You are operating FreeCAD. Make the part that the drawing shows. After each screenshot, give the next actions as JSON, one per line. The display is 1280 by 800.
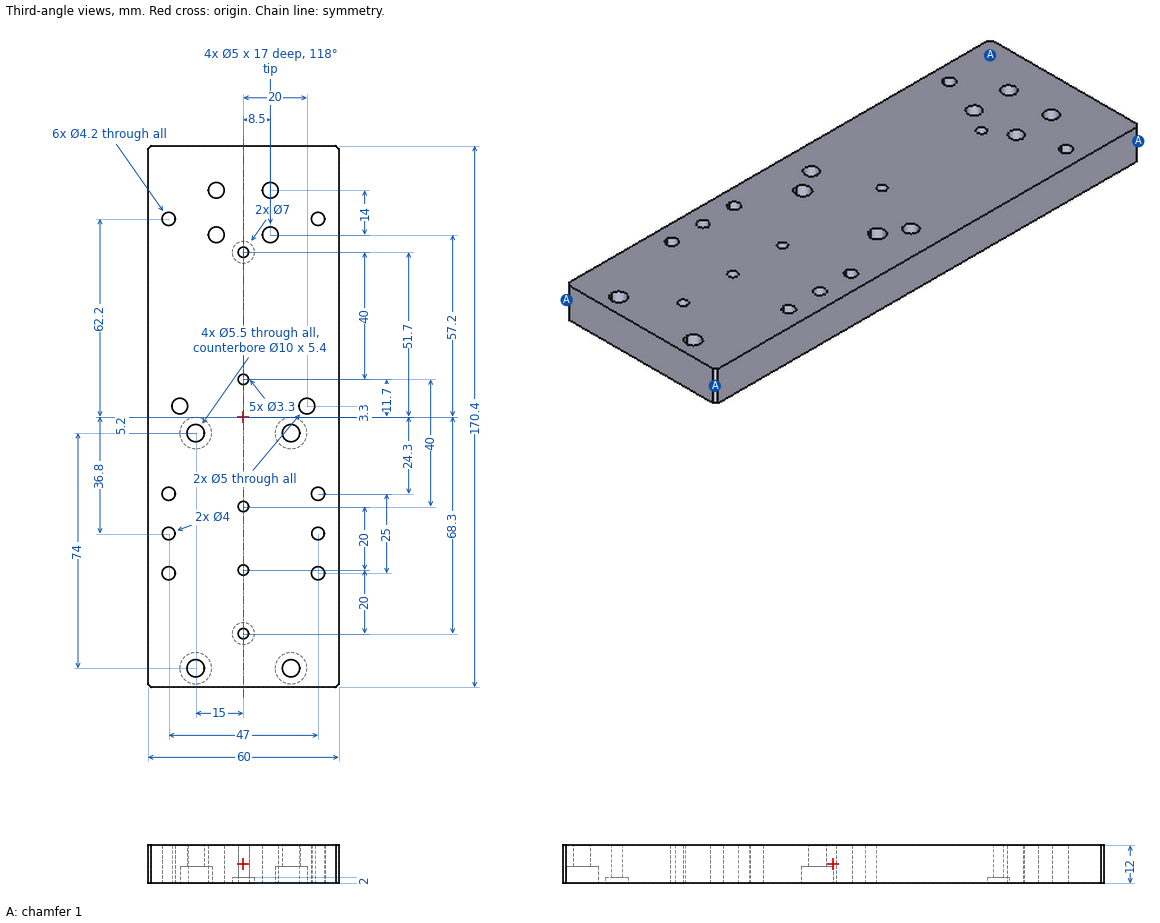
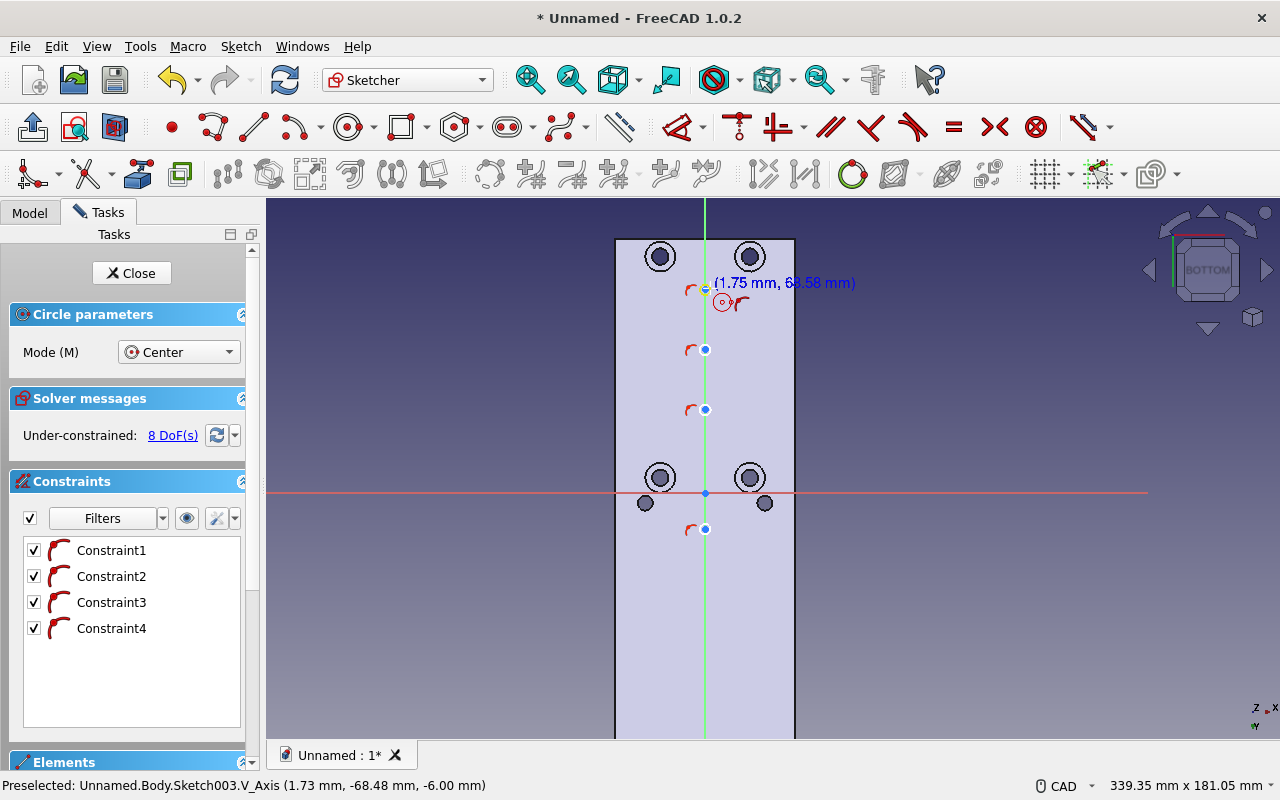
{"action": "scroll", "coordinate": [705, 648], "scroll_direction": "up", "scroll_amount": 8}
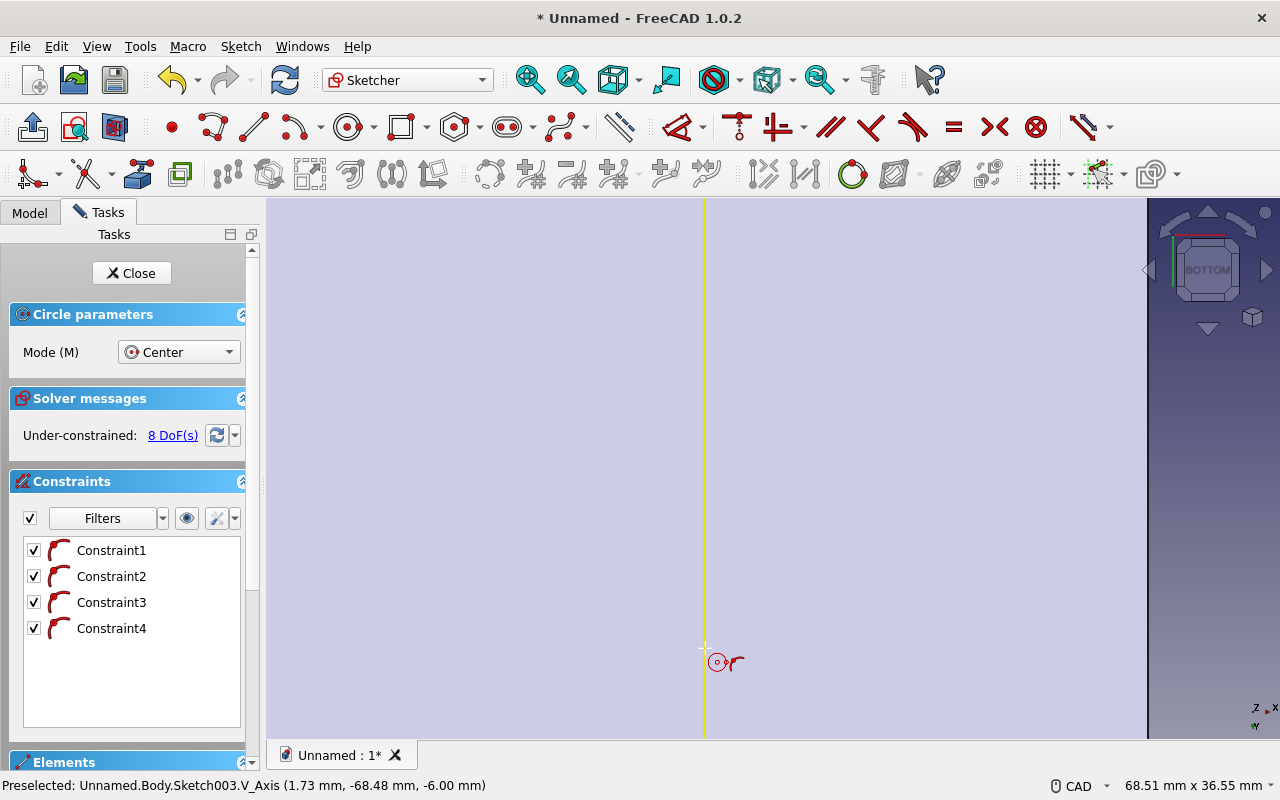
{"action": "scroll", "coordinate": [705, 649], "scroll_direction": "down", "scroll_amount": 8}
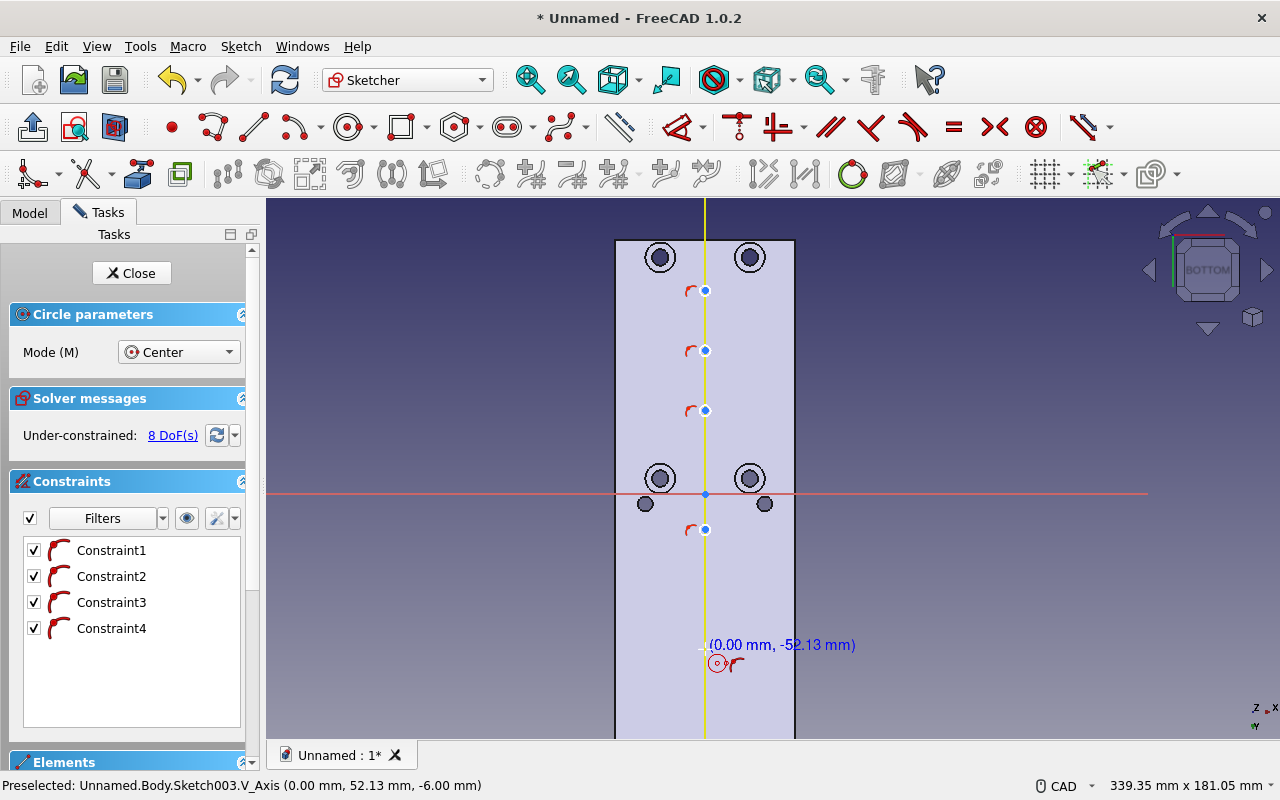
{"action": "left_click", "coordinate": [705, 649]}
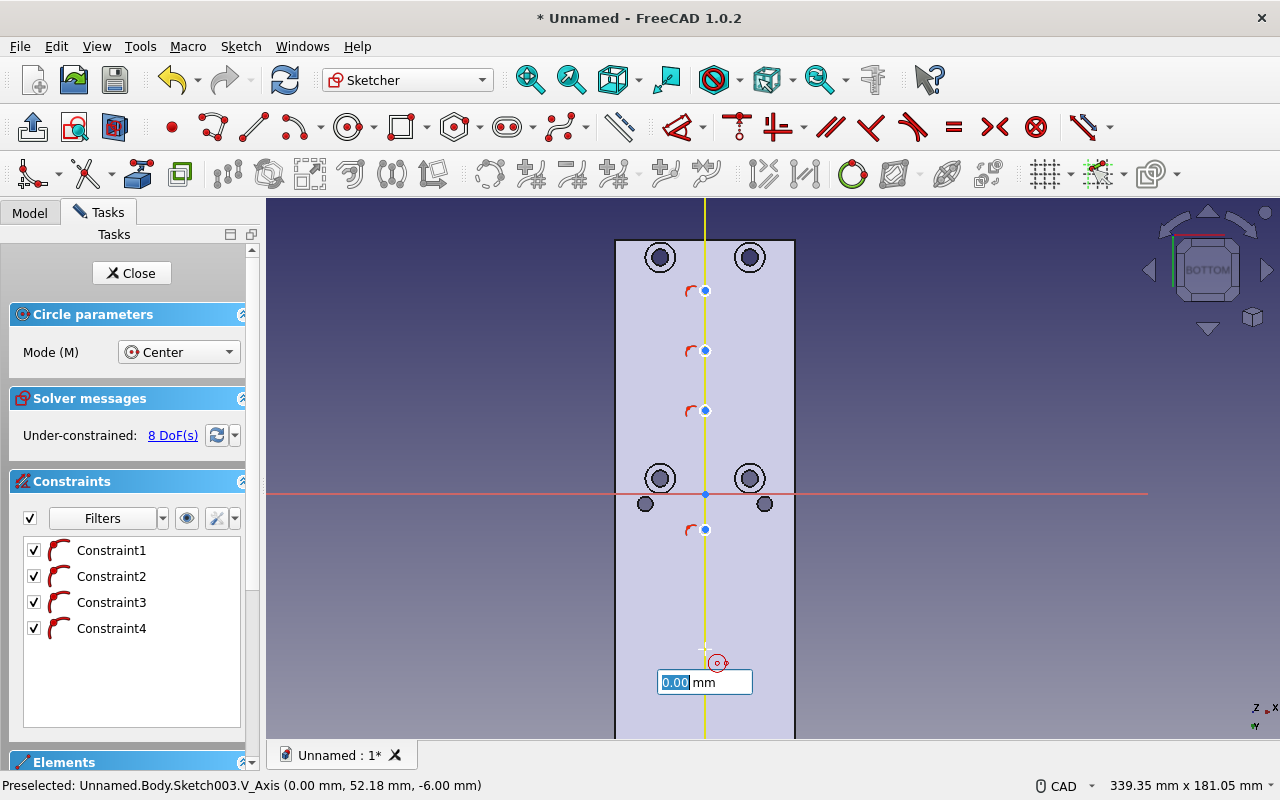
{"action": "scroll", "coordinate": [710, 647], "scroll_direction": "up", "scroll_amount": 7}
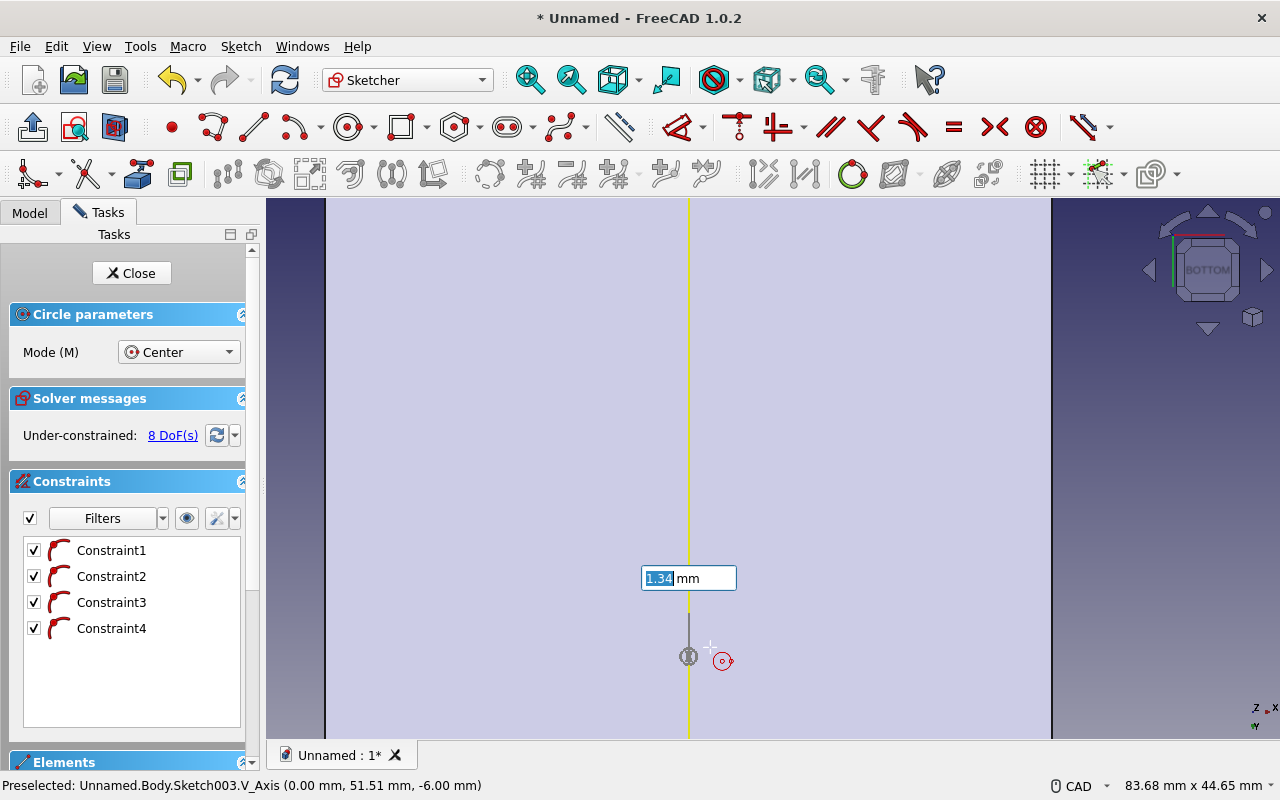
{"action": "left_click", "coordinate": [708, 644]}
{"action": "key", "text": "Escape"}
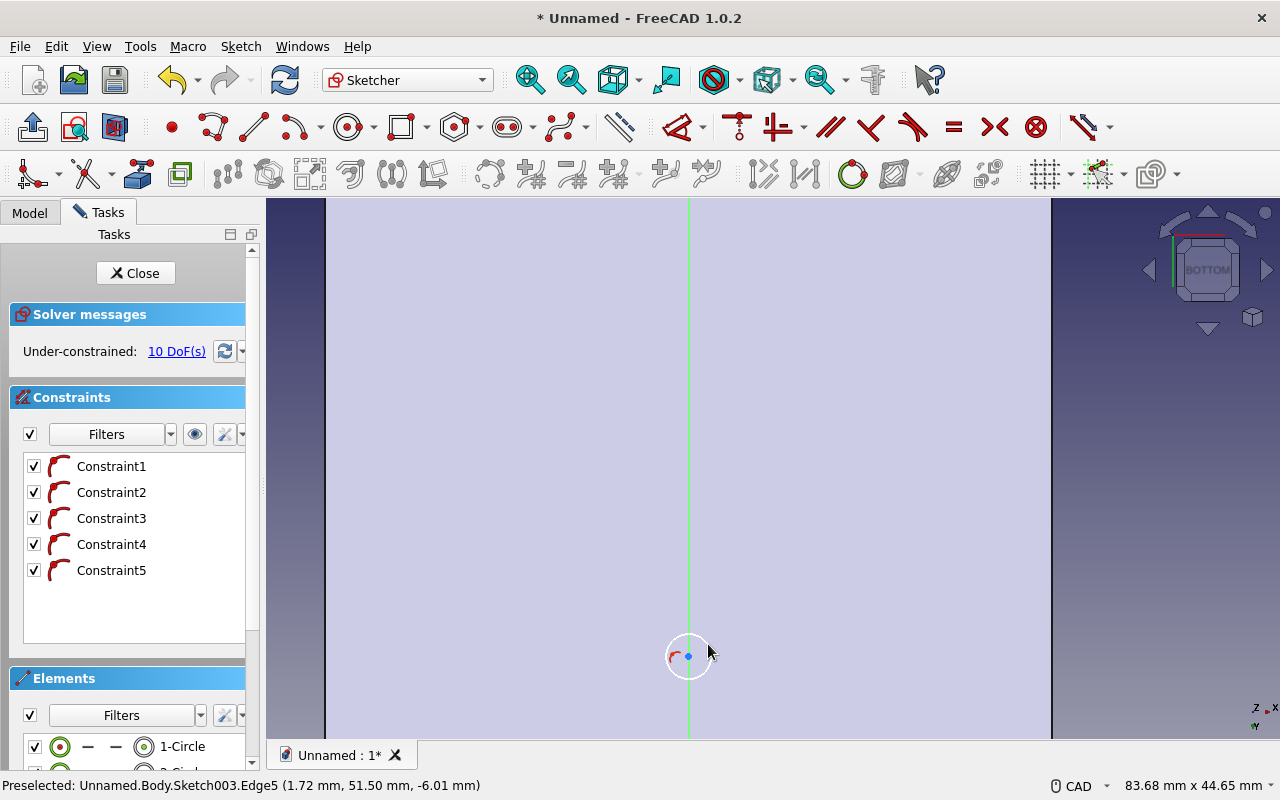
{"action": "scroll", "coordinate": [710, 647], "scroll_direction": "down", "scroll_amount": 7}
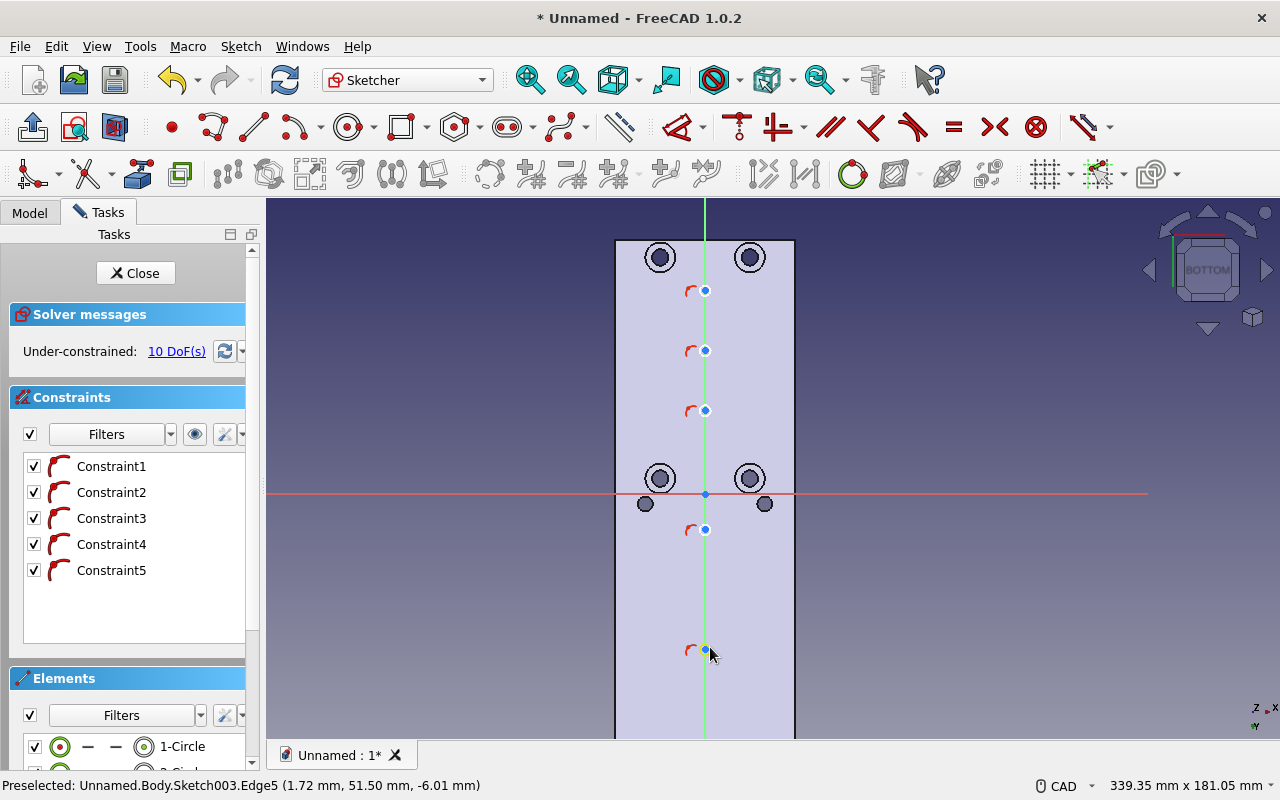
{"action": "scroll", "coordinate": [709, 526], "scroll_direction": "up", "scroll_amount": 7}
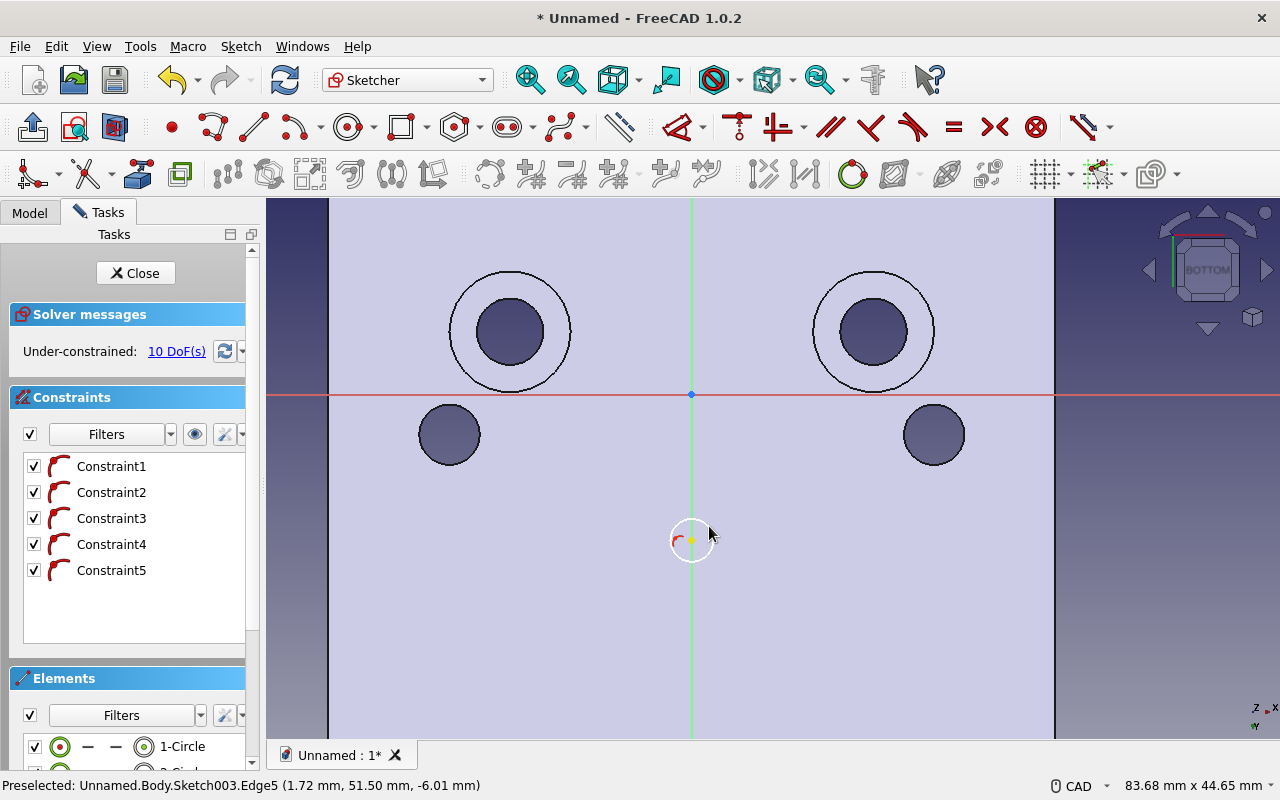
{"action": "left_click", "coordinate": [707, 525]}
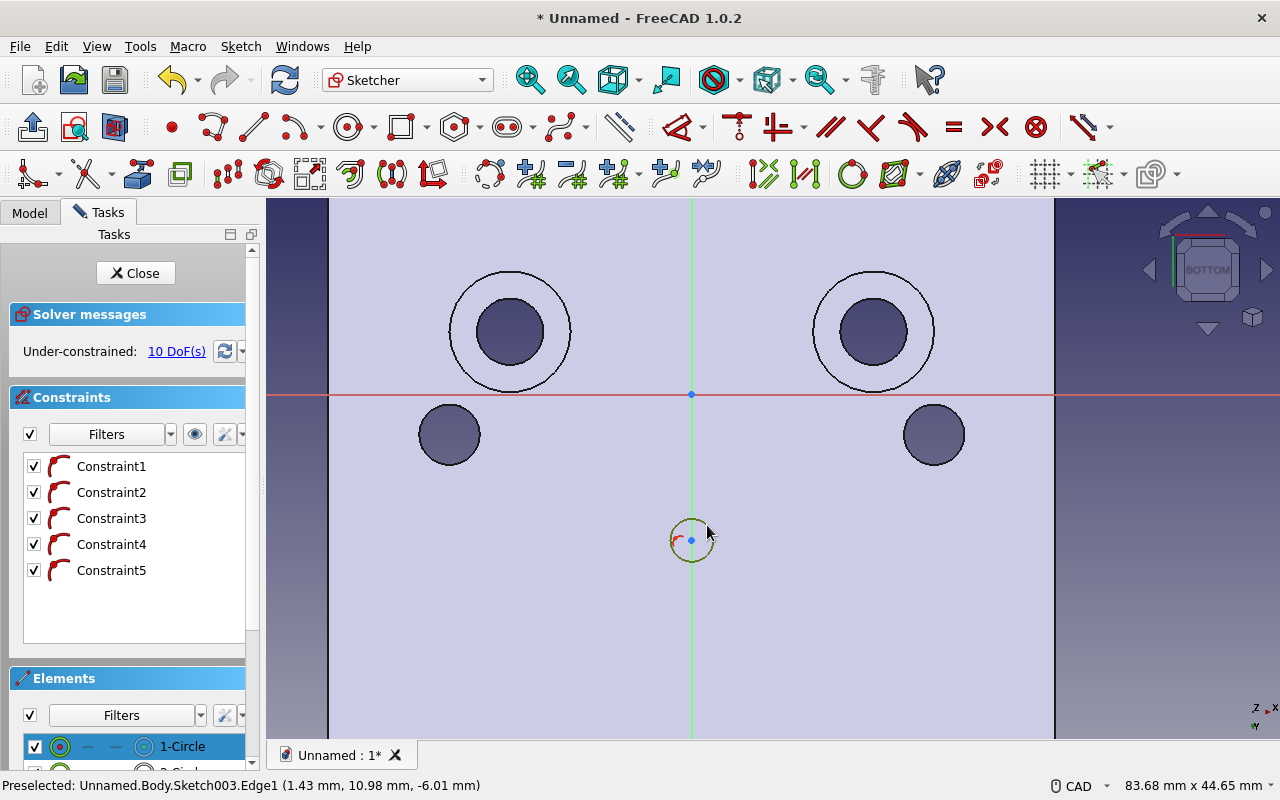
{"action": "scroll", "coordinate": [709, 526], "scroll_direction": "down", "scroll_amount": 7}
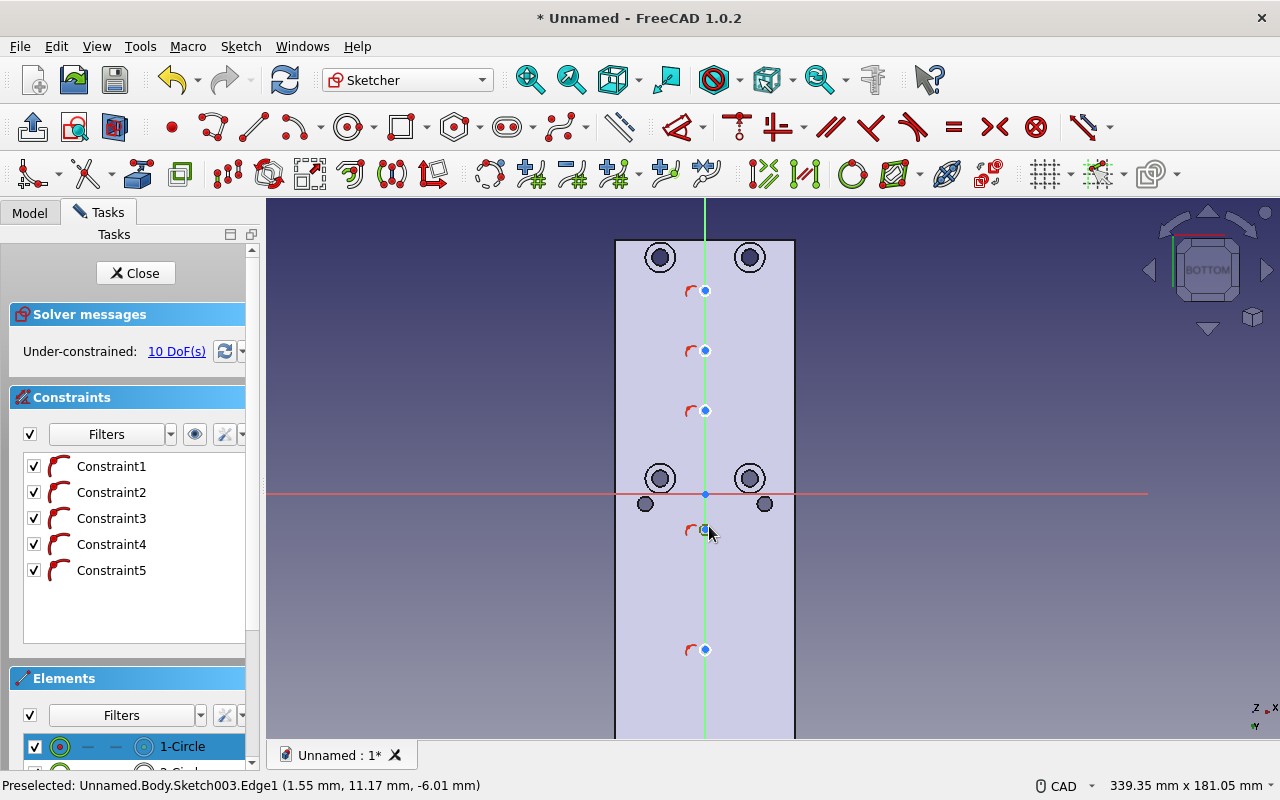
{"action": "scroll", "coordinate": [709, 407], "scroll_direction": "up", "scroll_amount": 7}